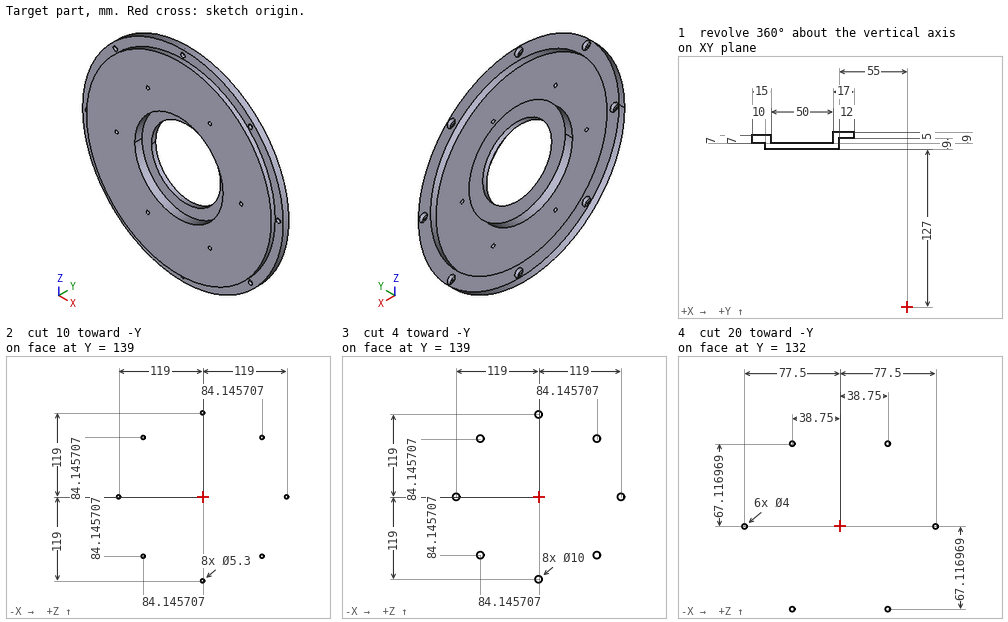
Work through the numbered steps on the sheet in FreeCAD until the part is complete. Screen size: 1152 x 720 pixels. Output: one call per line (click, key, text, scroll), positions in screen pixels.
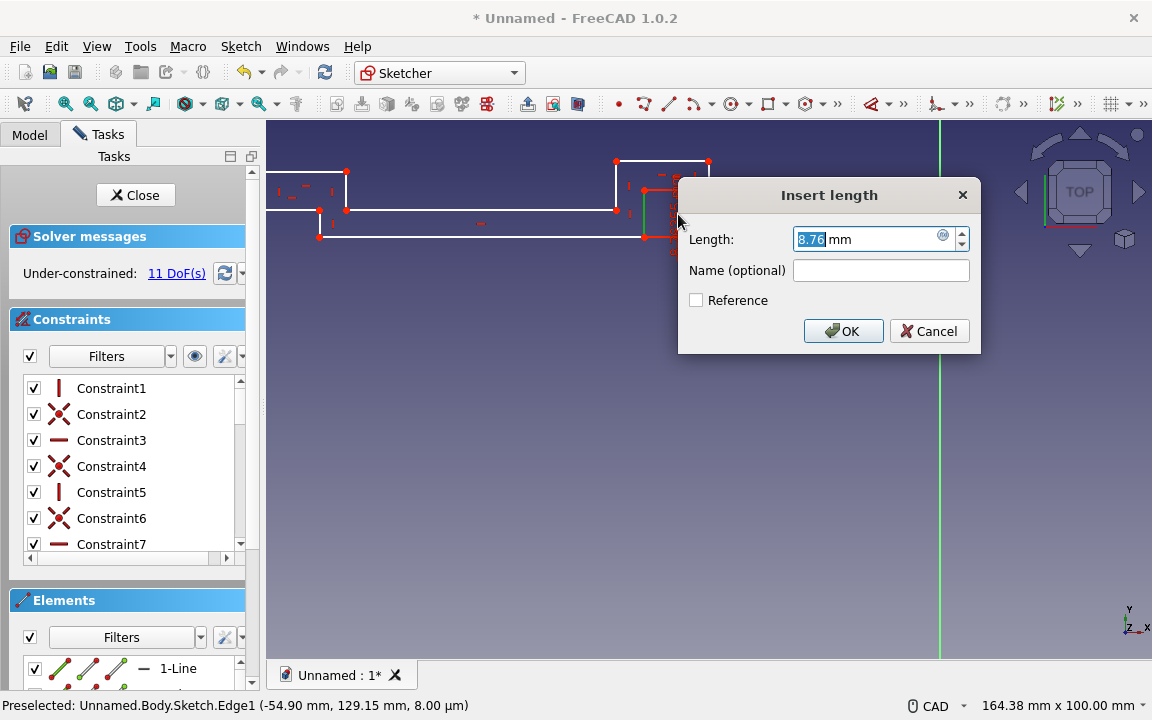
text(9)
key(Return)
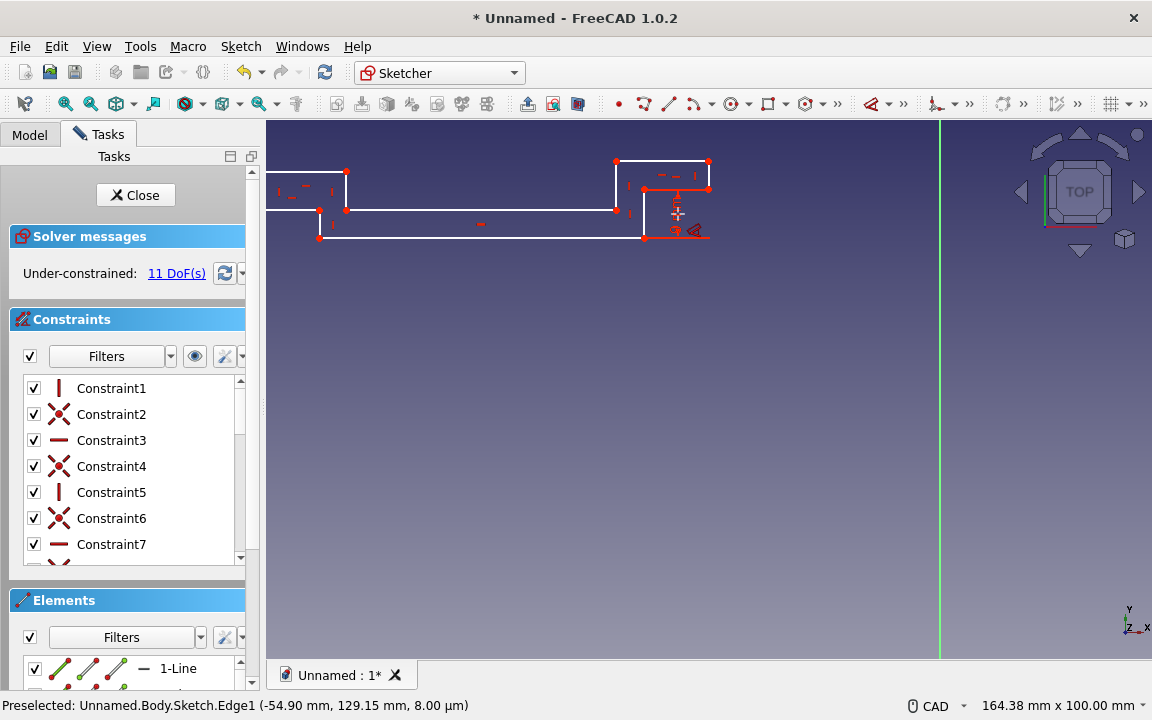
scroll(709, 178, up, 2)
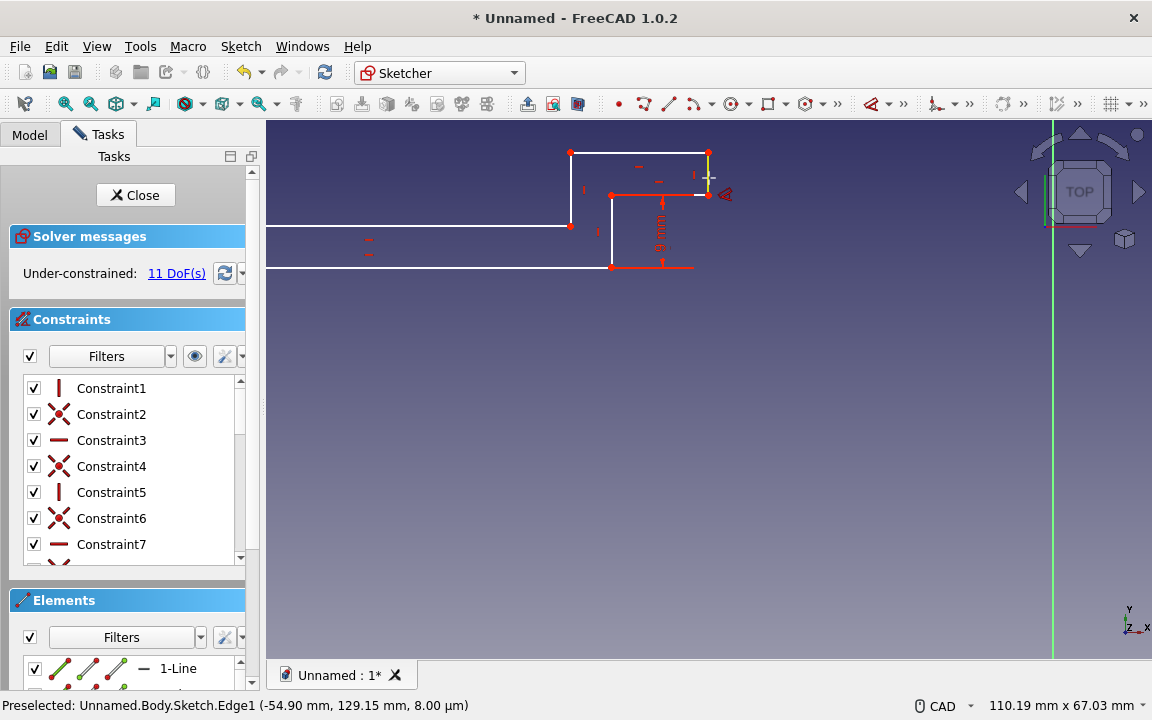
click(708, 178)
click(742, 174)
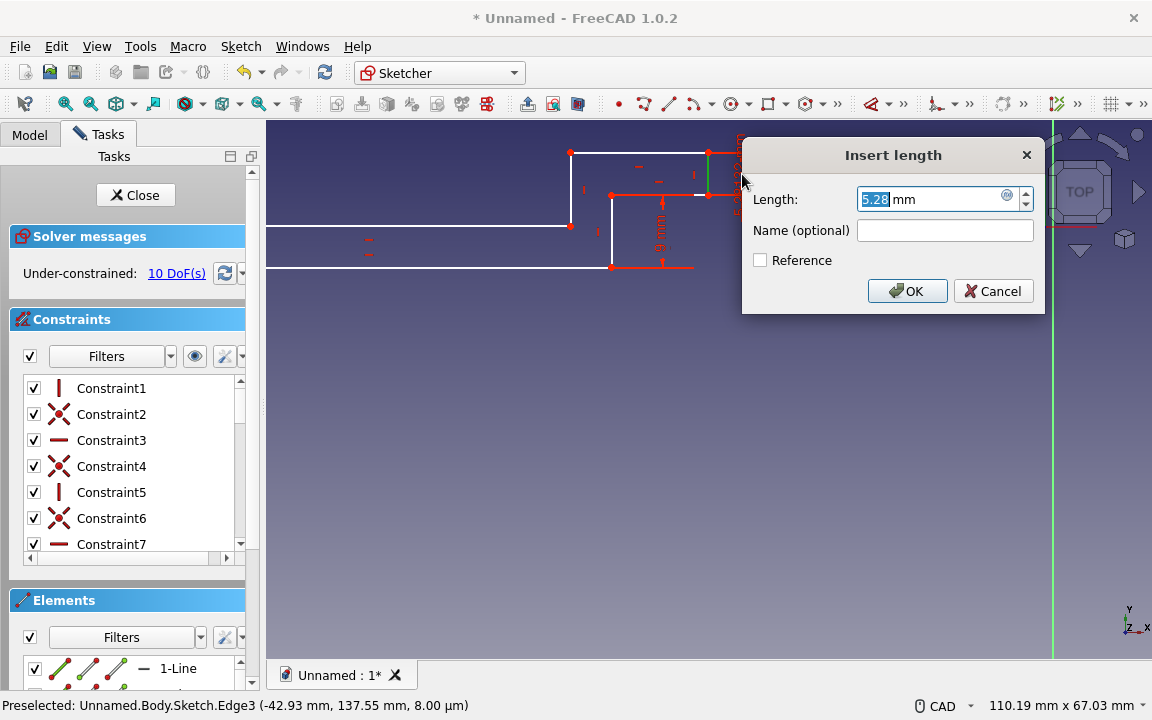
text(5)
key(Return)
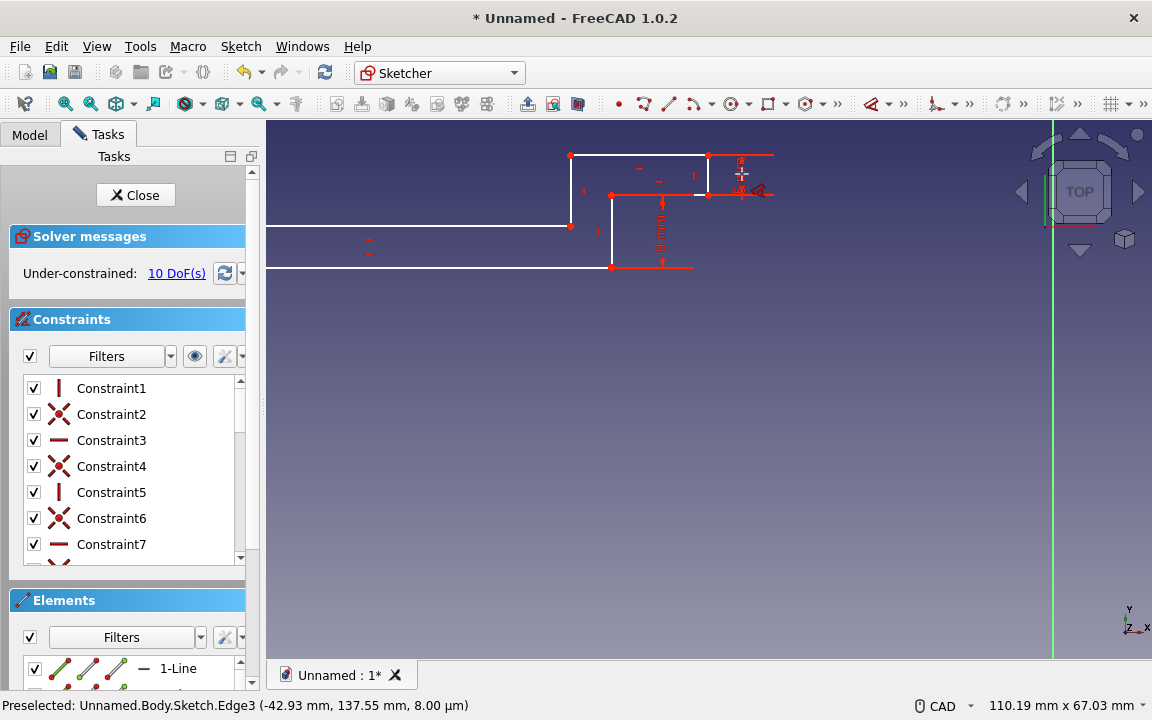
click(571, 177)
click(605, 174)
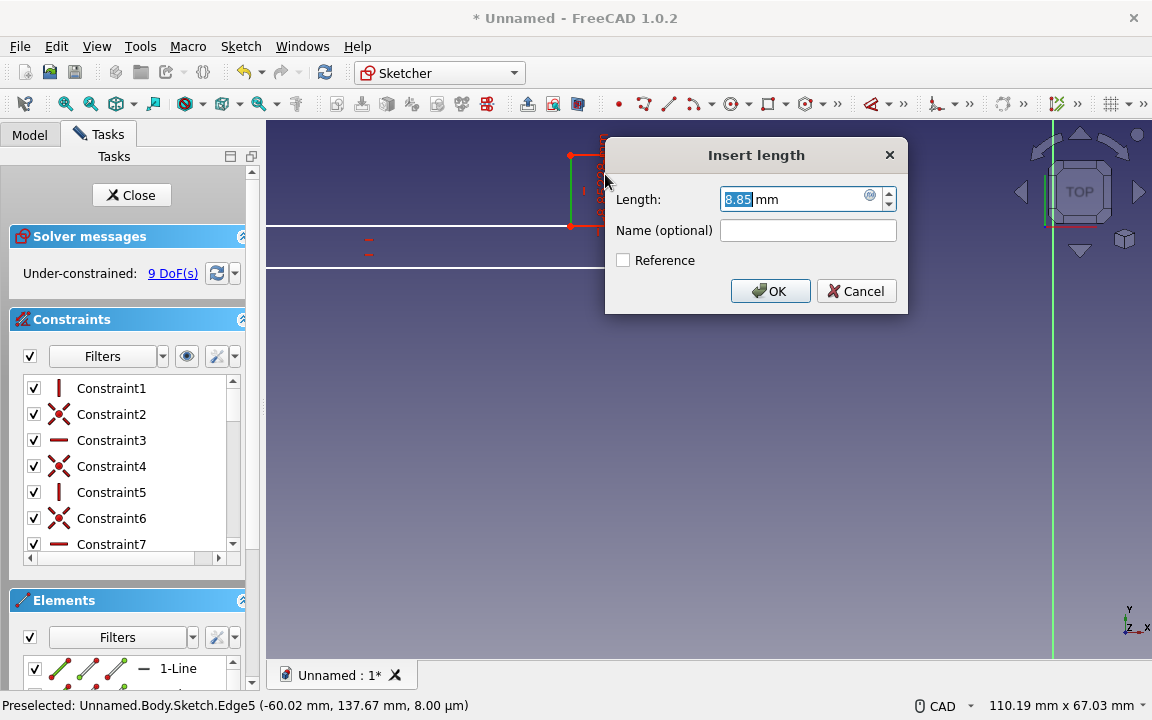
text(9)
key(Return)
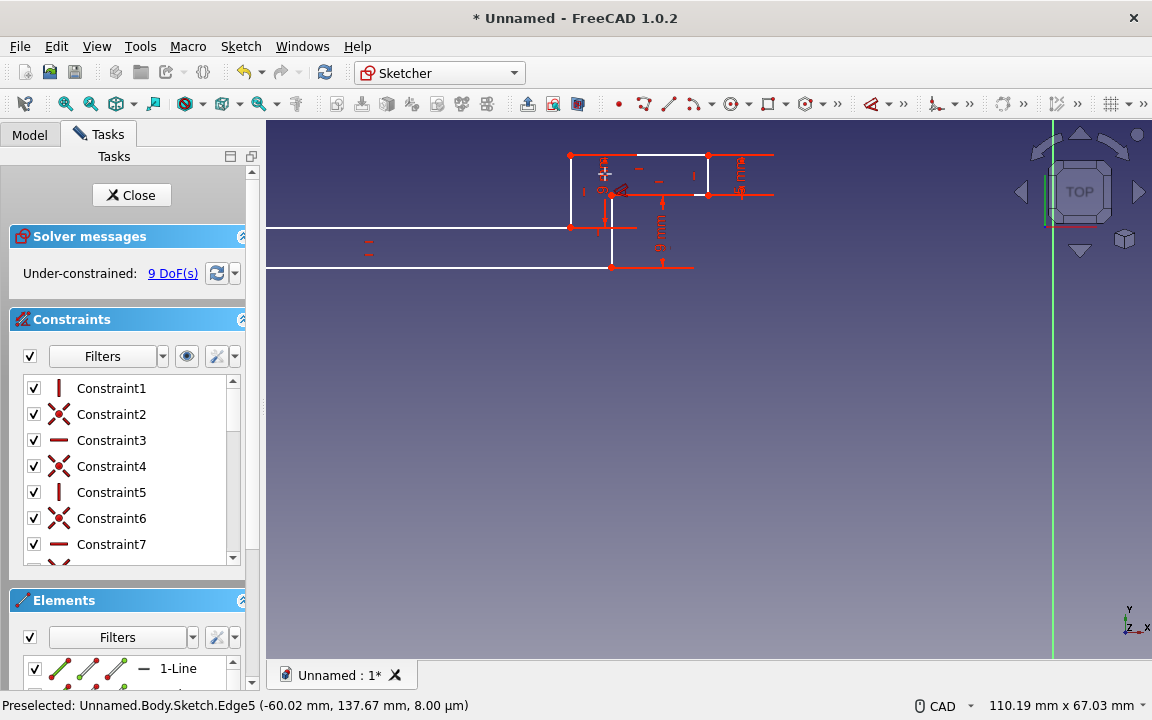
scroll(679, 248, down, 6)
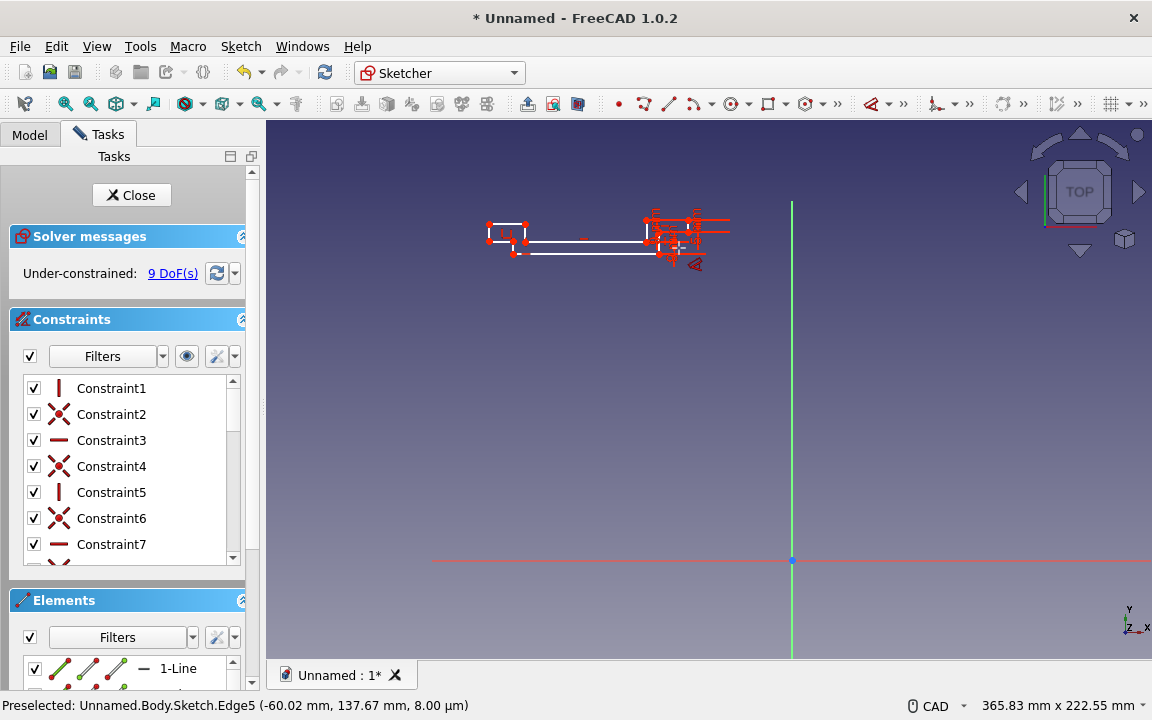
scroll(525, 237, up, 5)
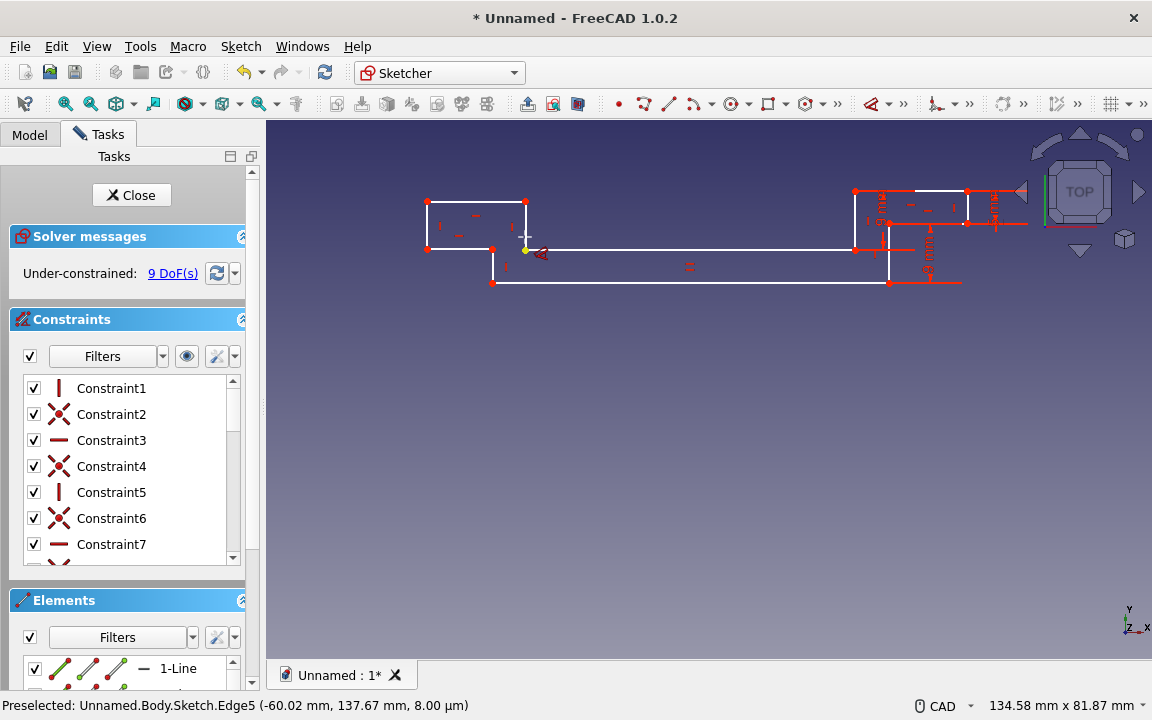
click(526, 236)
click(492, 226)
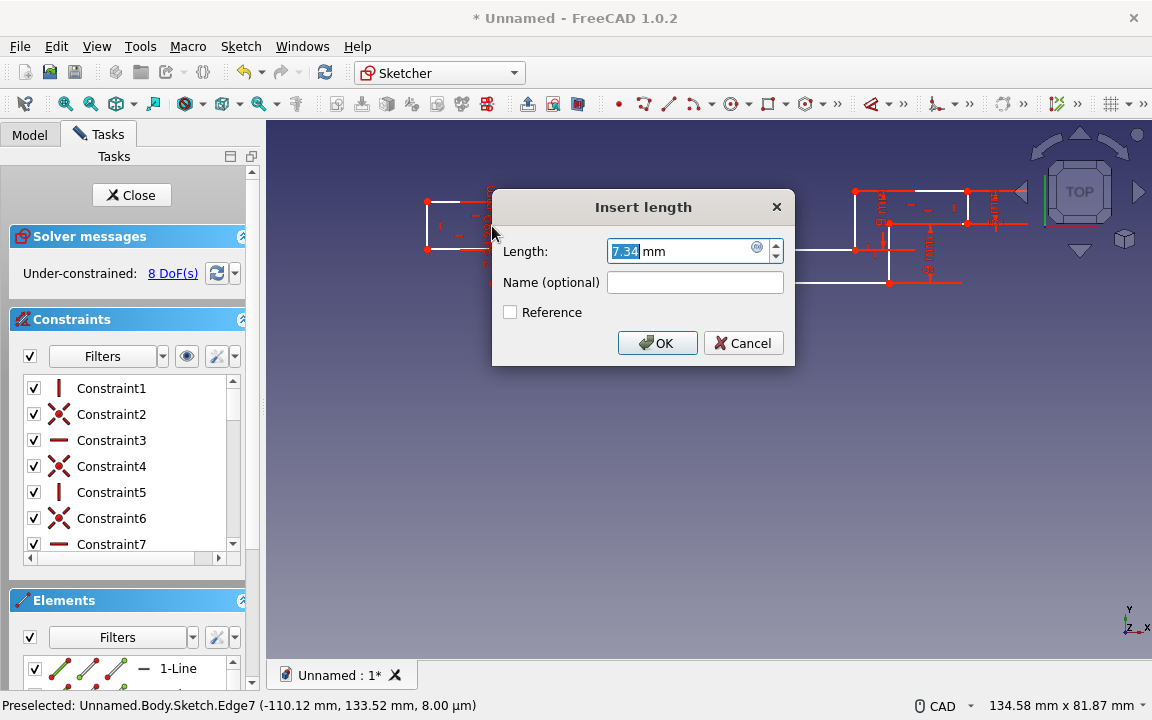
text(7)
key(Return)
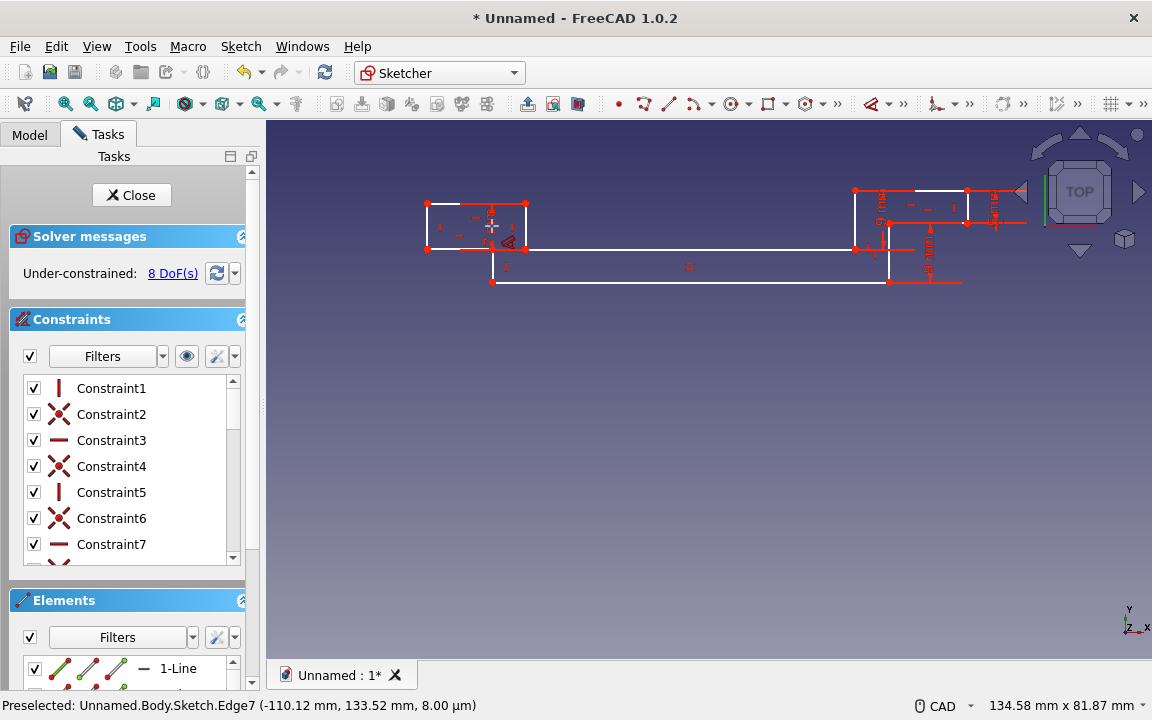
click(427, 217)
click(393, 227)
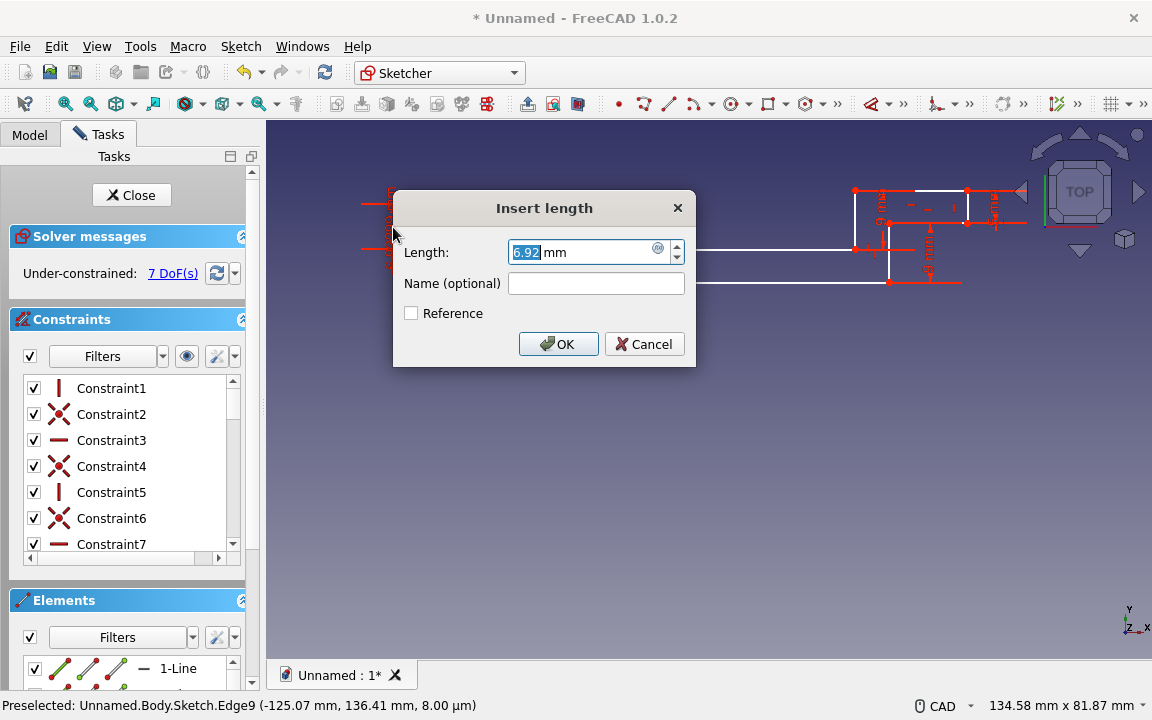
text(7)
key(Return)